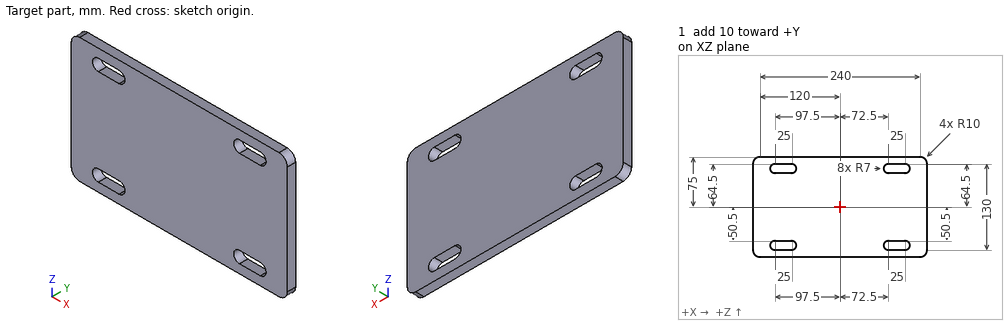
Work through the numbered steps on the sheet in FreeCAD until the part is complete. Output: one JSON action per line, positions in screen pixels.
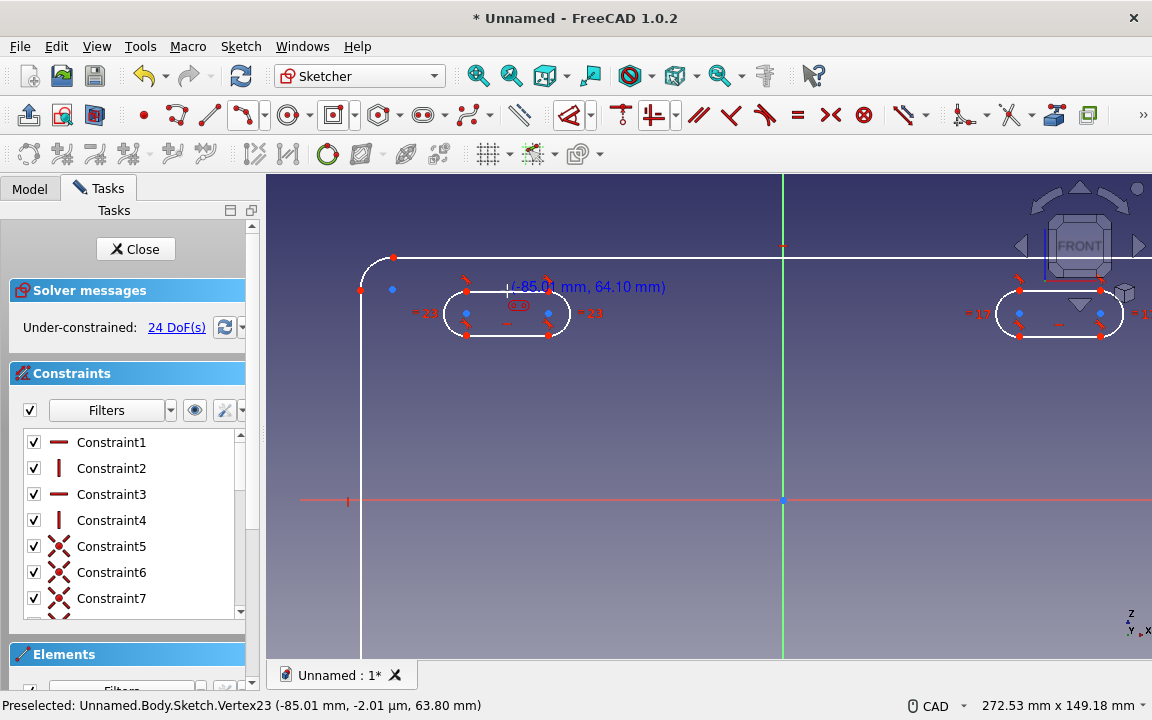
{"action": "scroll", "coordinate": [467, 314], "scroll_direction": "down", "scroll_amount": 3}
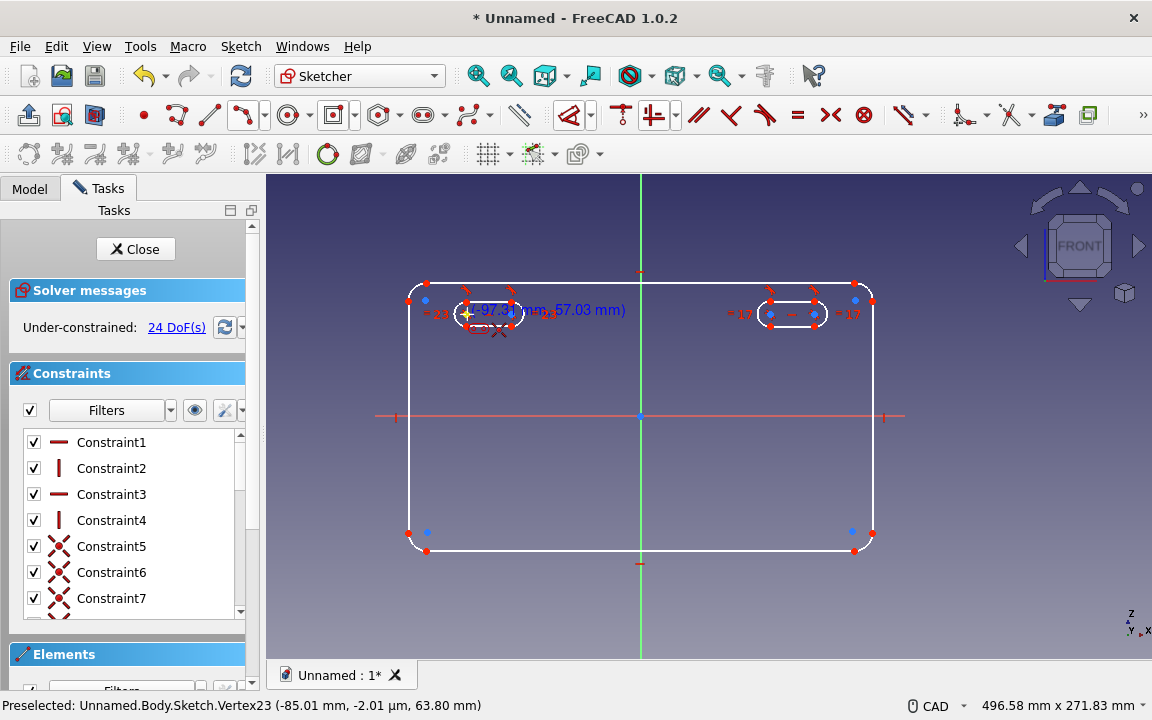
{"action": "scroll", "coordinate": [770, 519], "scroll_direction": "up", "scroll_amount": 3}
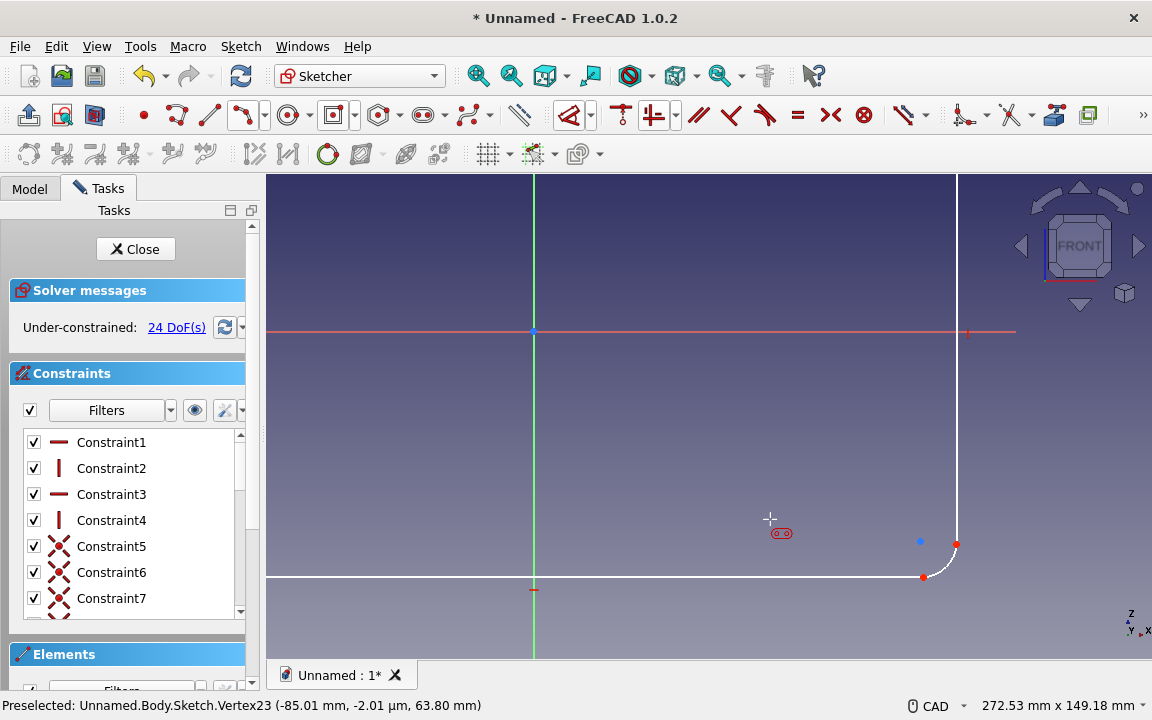
{"action": "left_click", "coordinate": [770, 518]}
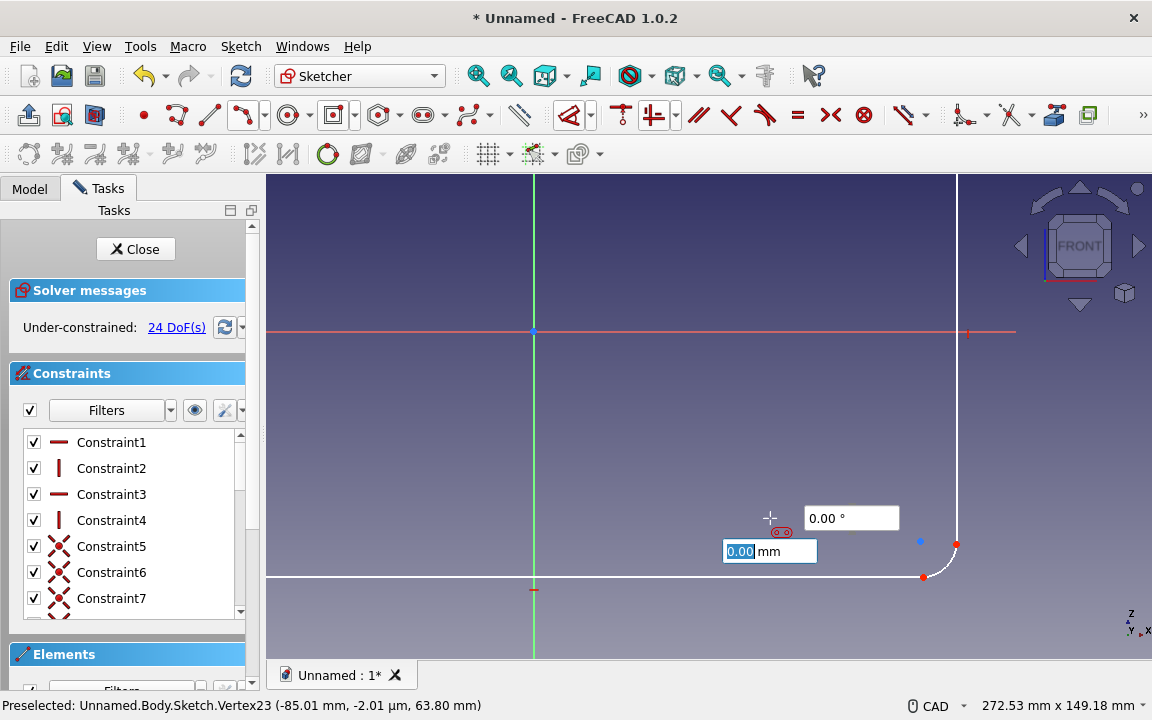
{"action": "left_click", "coordinate": [851, 518]}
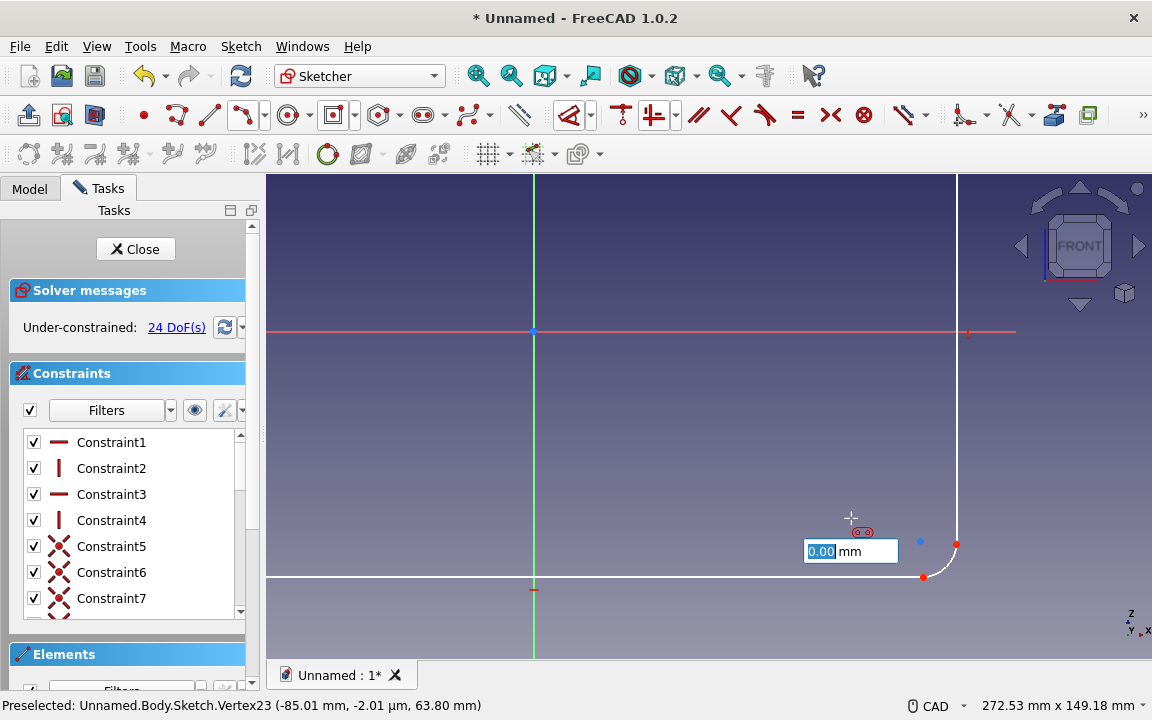
{"action": "left_click", "coordinate": [810, 541]}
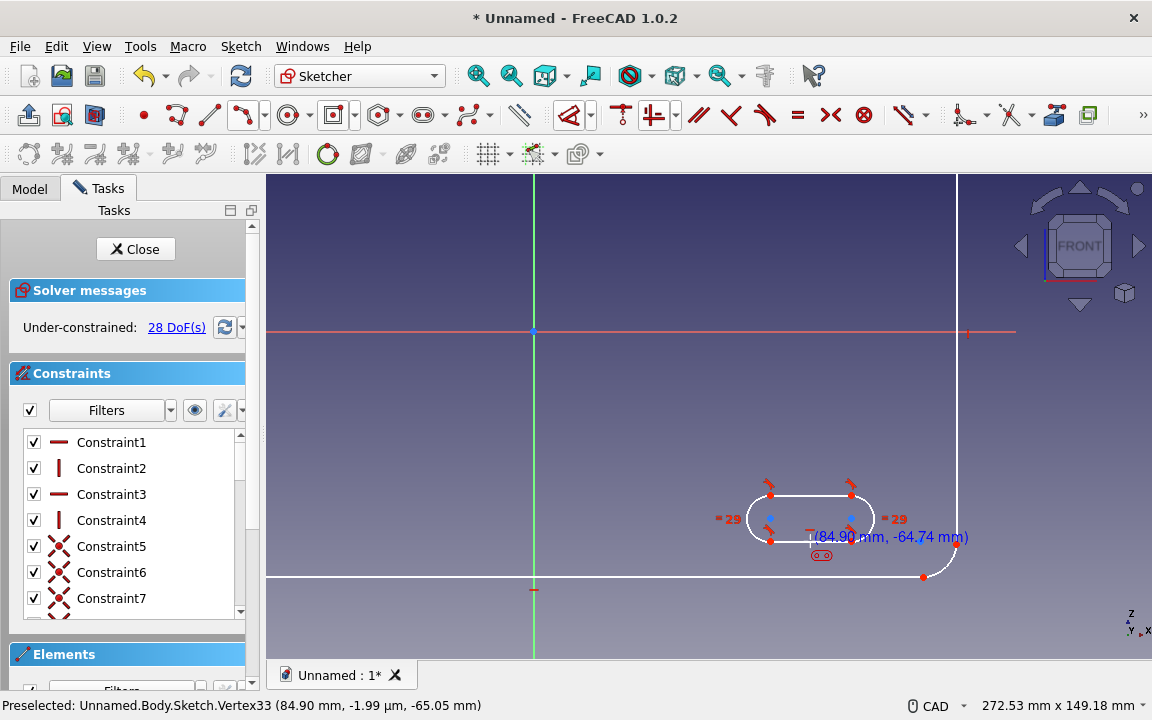
{"action": "scroll", "coordinate": [770, 520], "scroll_direction": "down", "scroll_amount": 3}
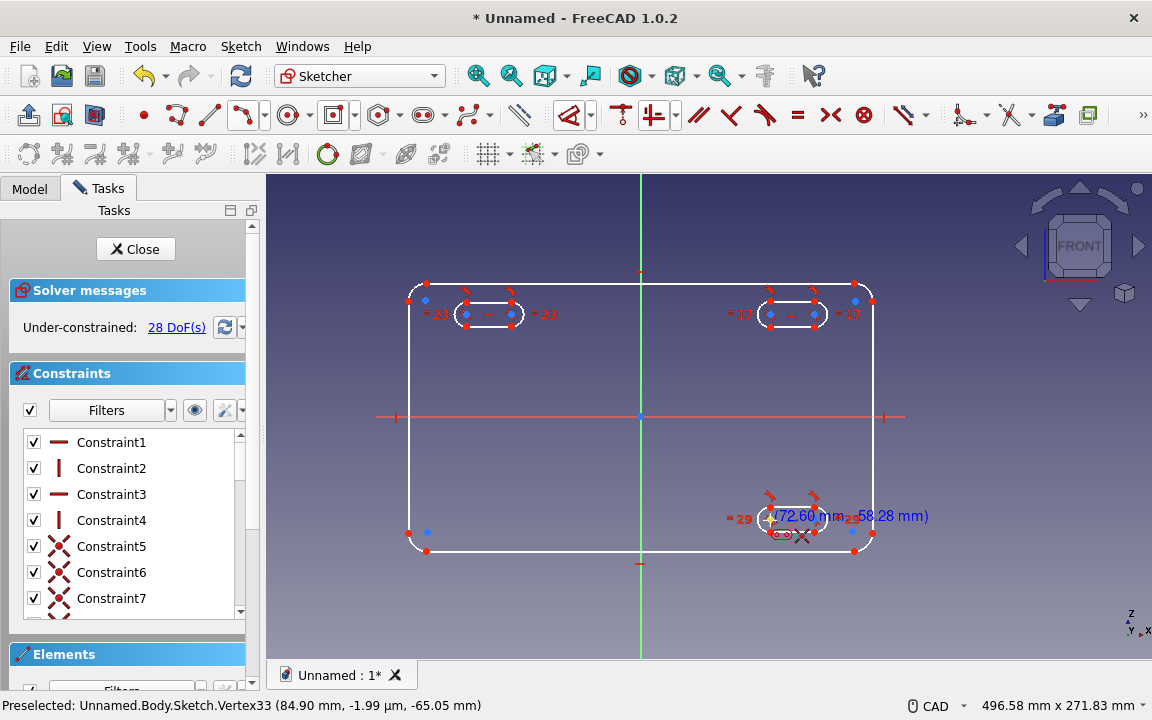
{"action": "scroll", "coordinate": [467, 519], "scroll_direction": "up", "scroll_amount": 3}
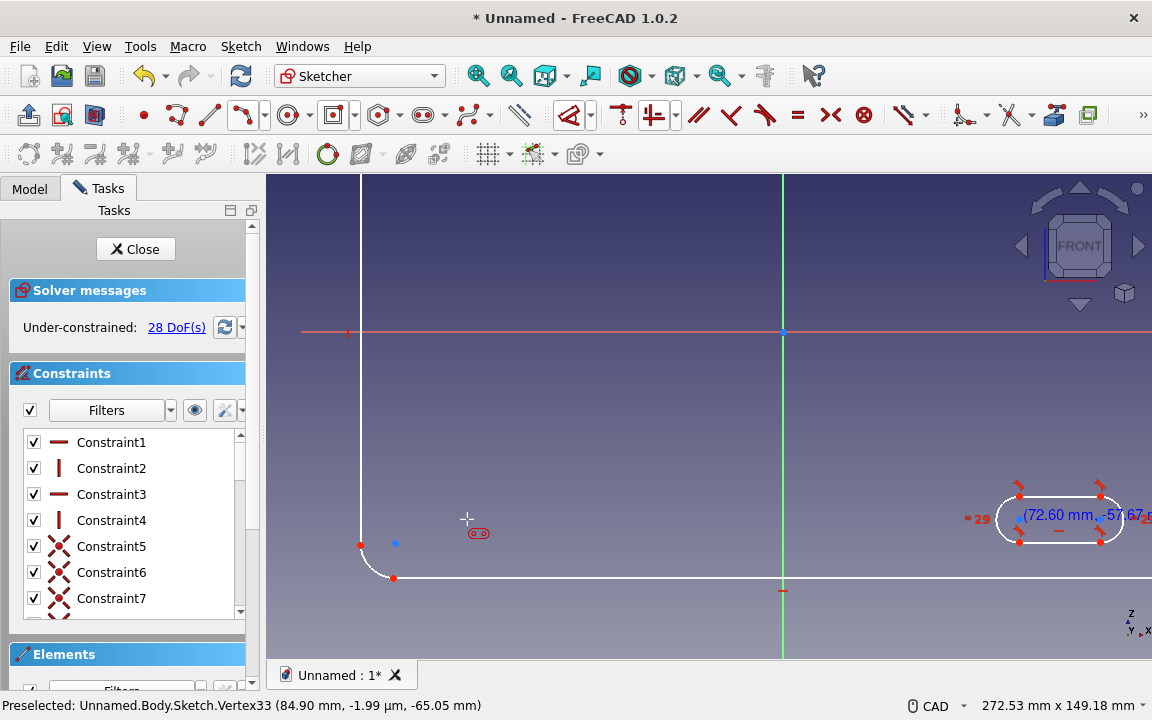
{"action": "left_click", "coordinate": [466, 519]}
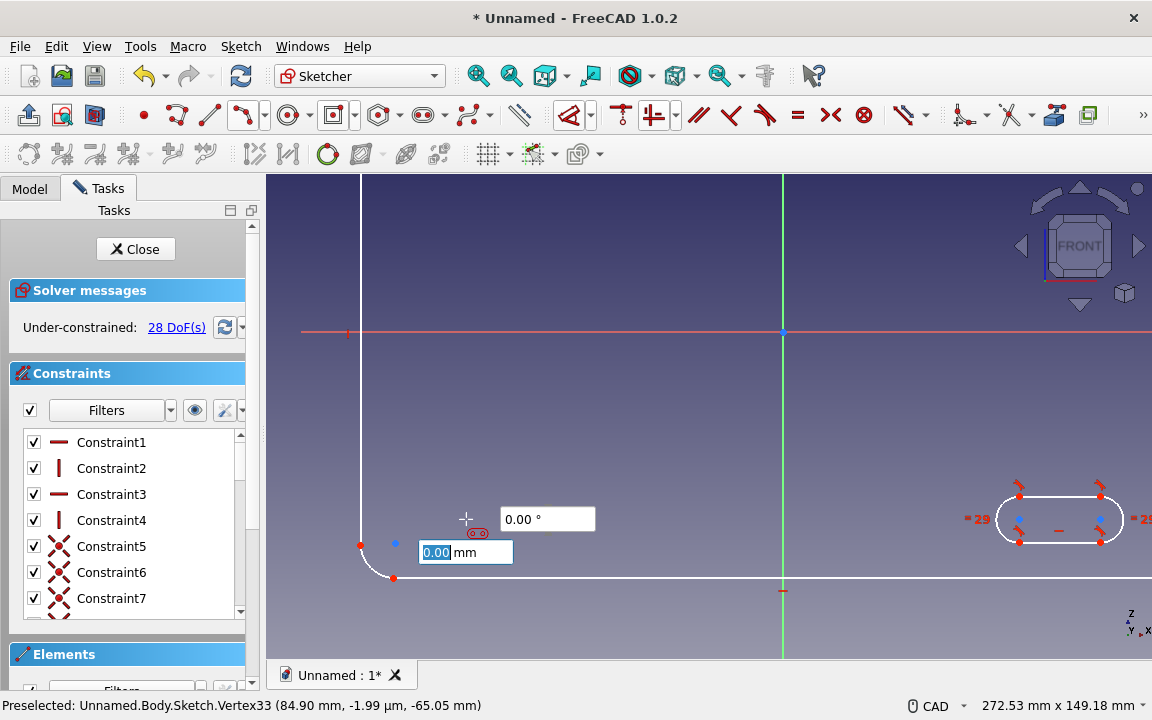
{"action": "left_click", "coordinate": [548, 519]}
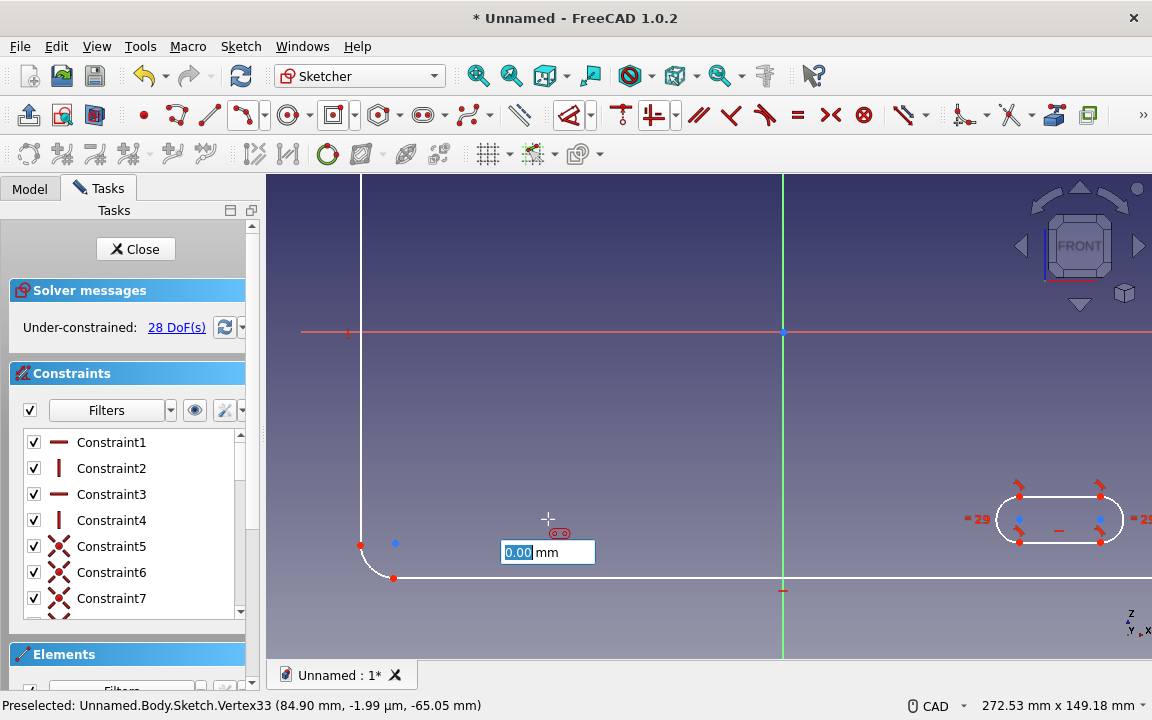
{"action": "left_click", "coordinate": [507, 497]}
{"action": "key", "text": "Escape"}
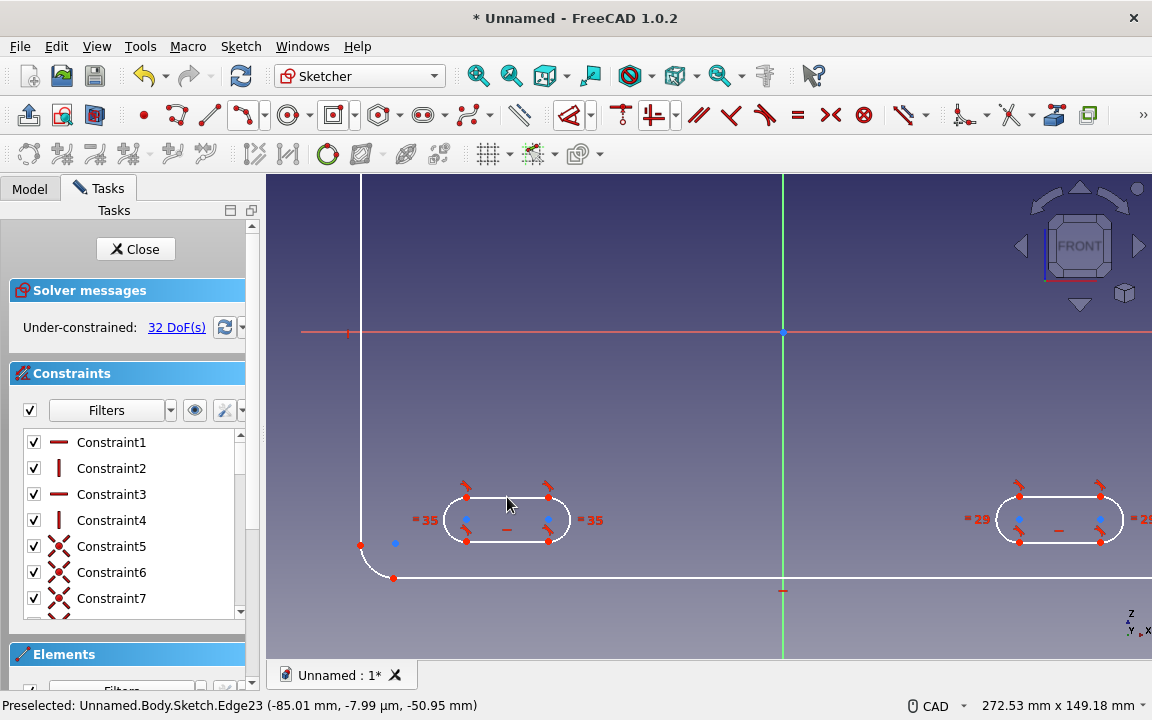
{"action": "scroll", "coordinate": [467, 519], "scroll_direction": "down", "scroll_amount": 3}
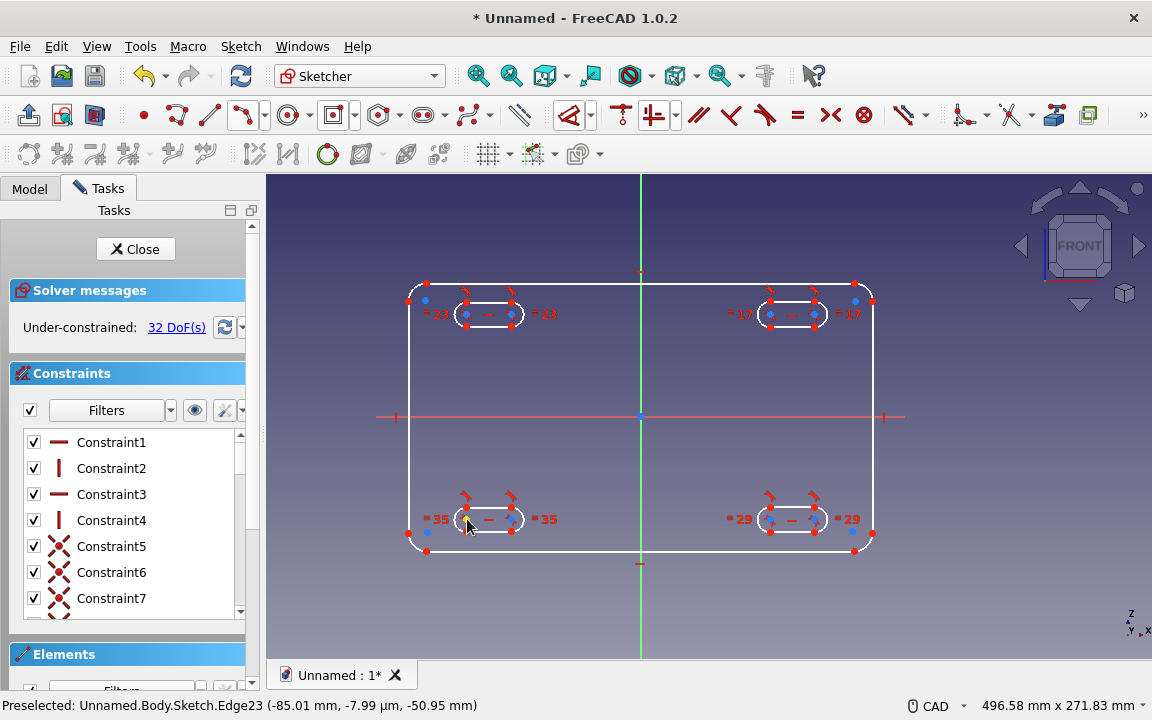
{"action": "left_click", "coordinate": [555, 284]}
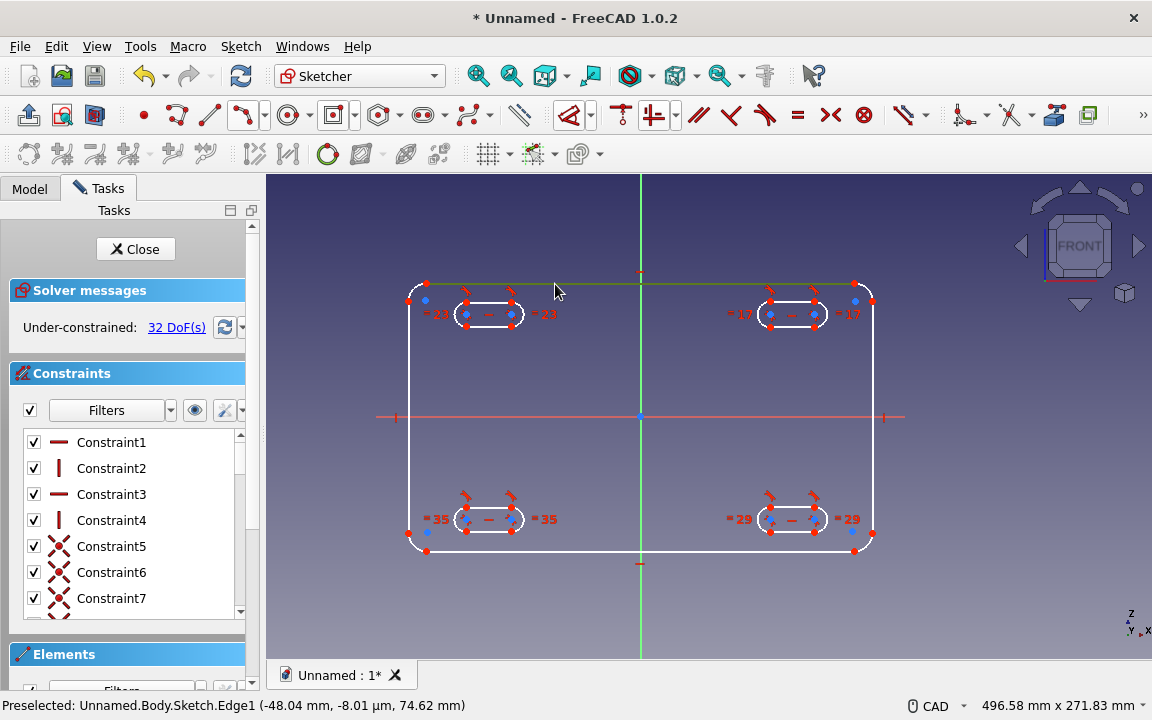
{"action": "left_click", "coordinate": [868, 289]}